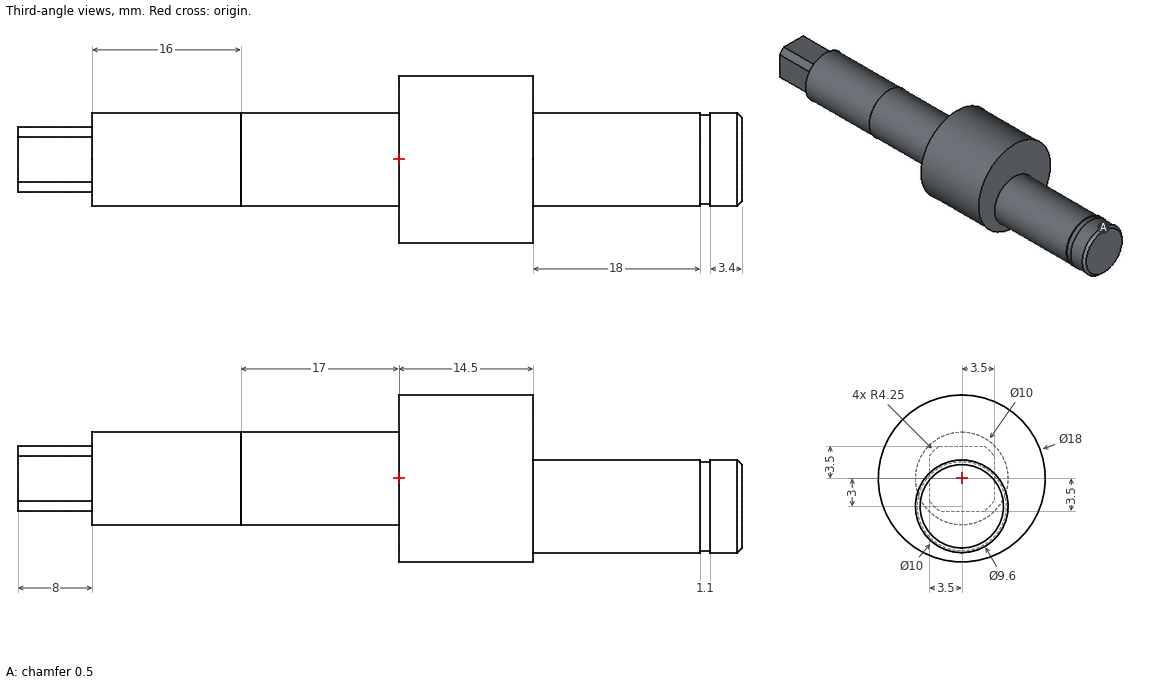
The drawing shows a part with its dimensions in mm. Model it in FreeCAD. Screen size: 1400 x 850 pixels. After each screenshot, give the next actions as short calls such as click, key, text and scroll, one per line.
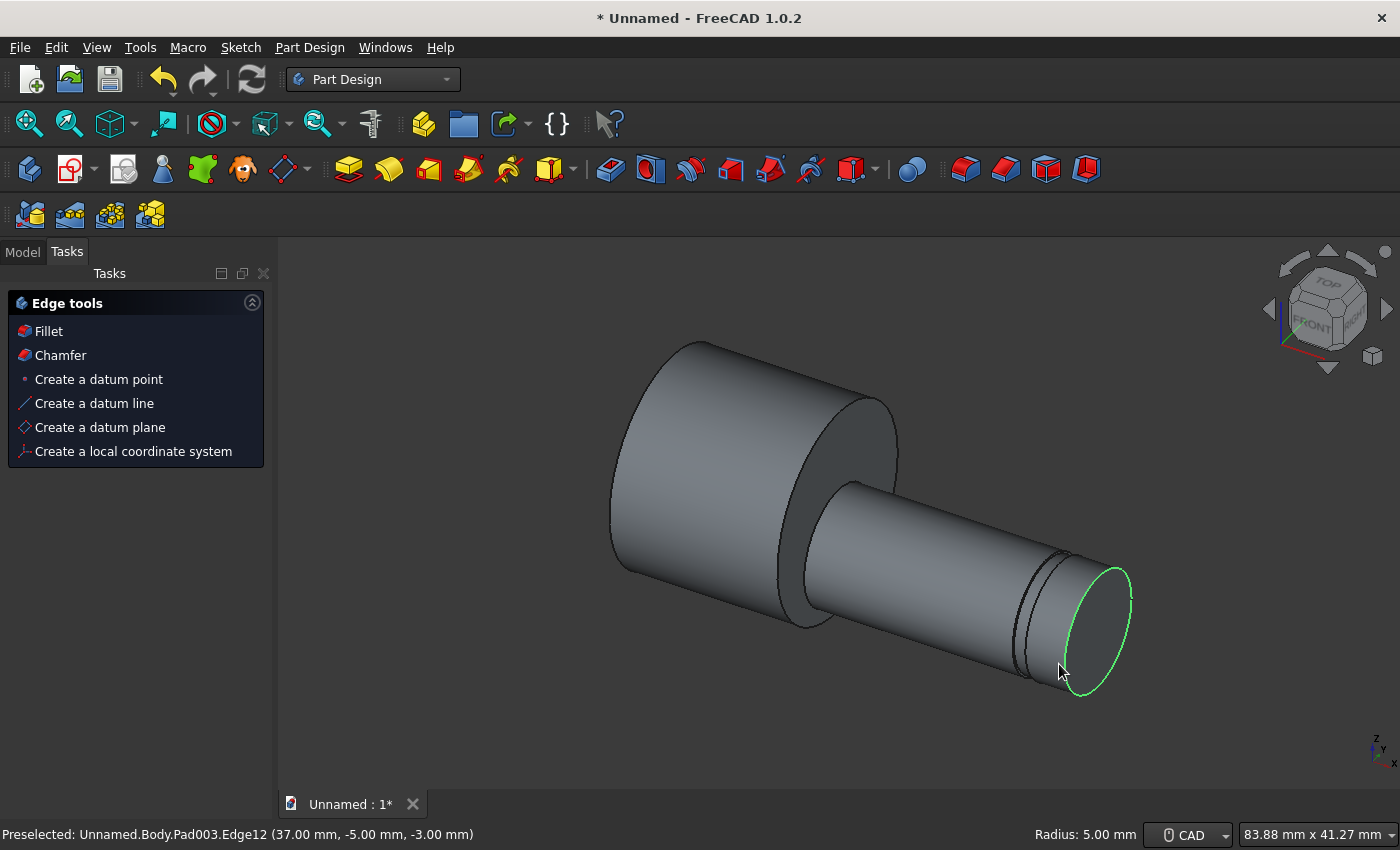
click(1006, 170)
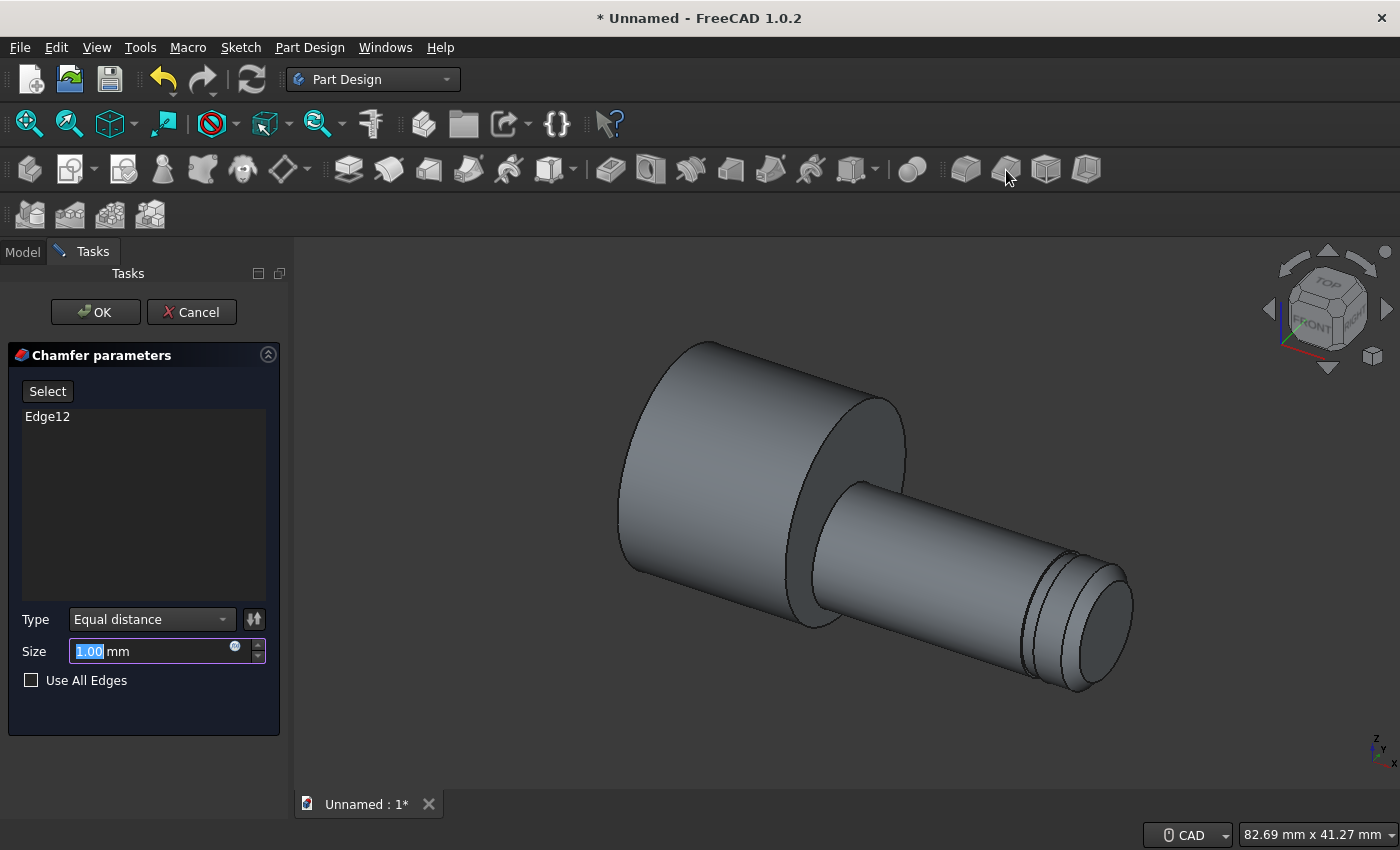
text(0.5)
key(Tab)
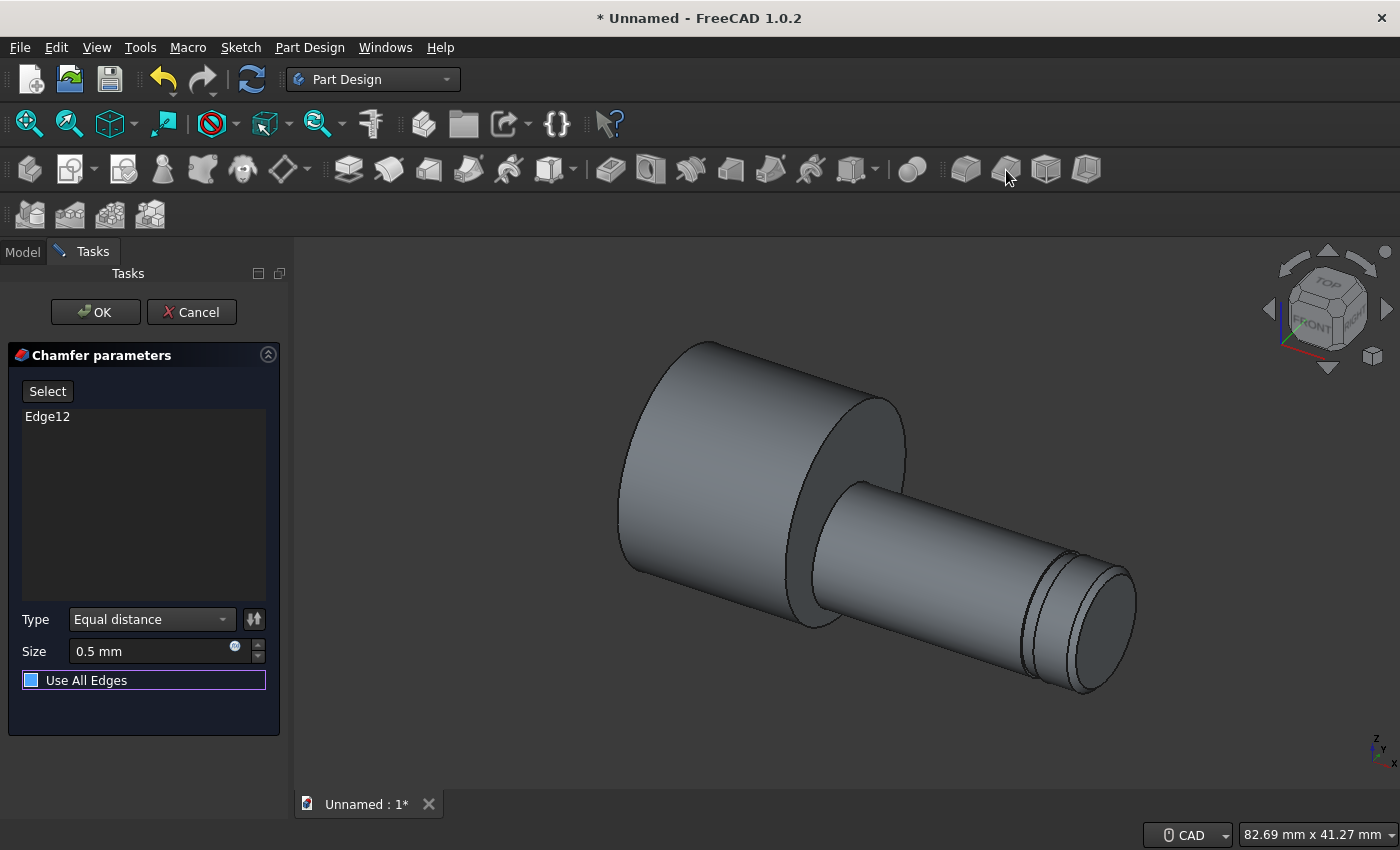
click(96, 312)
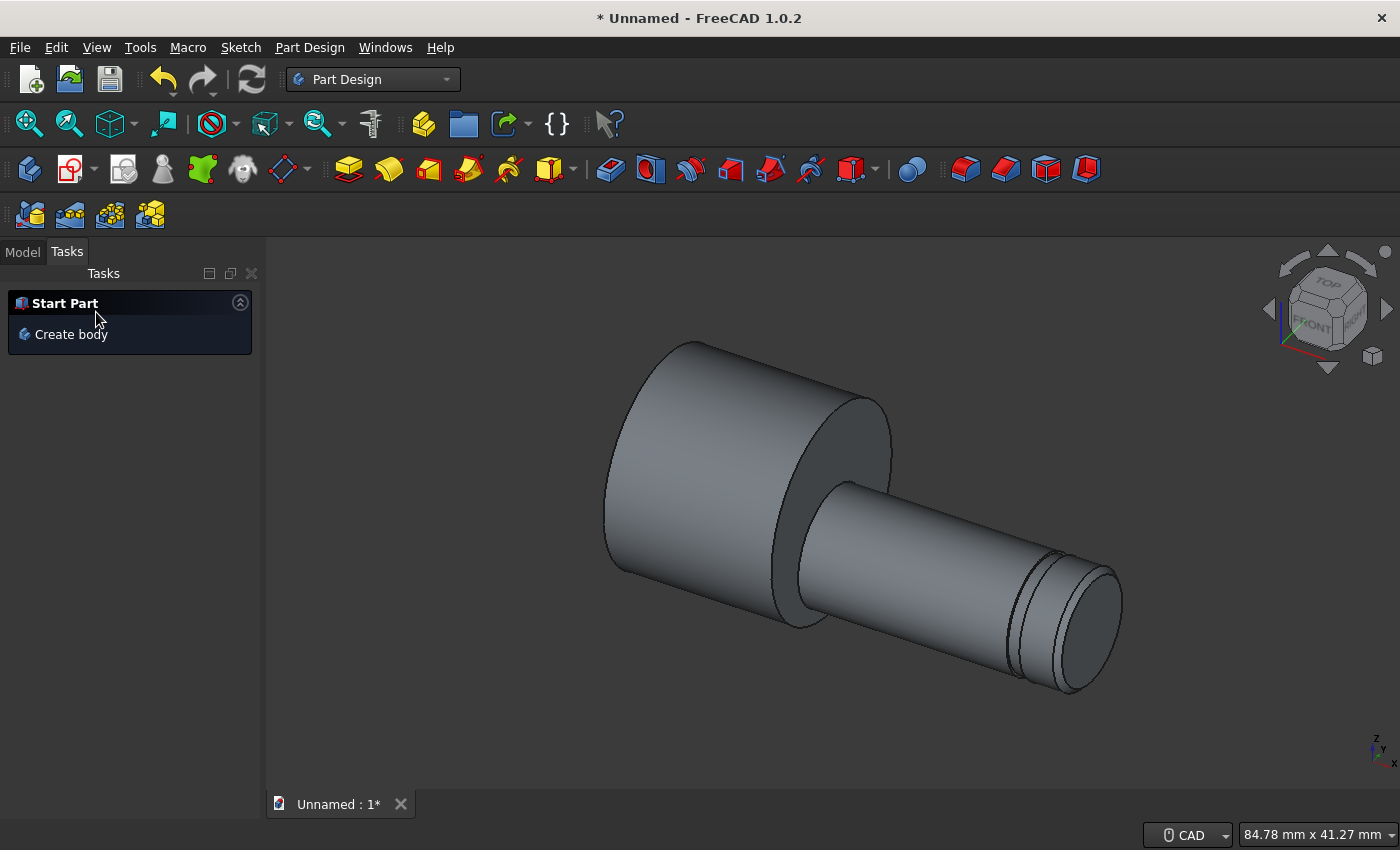
click(70, 170)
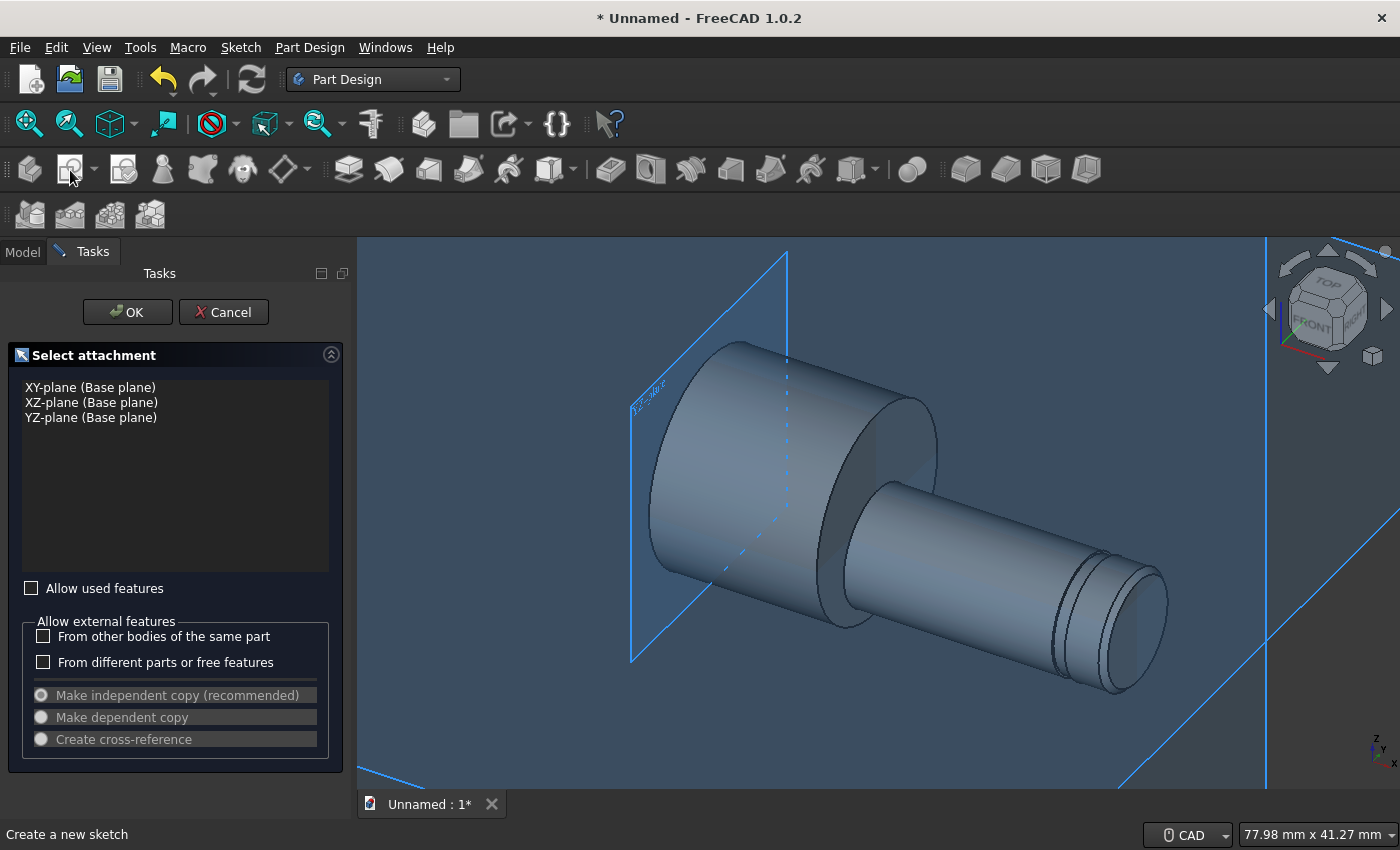
click(82, 418)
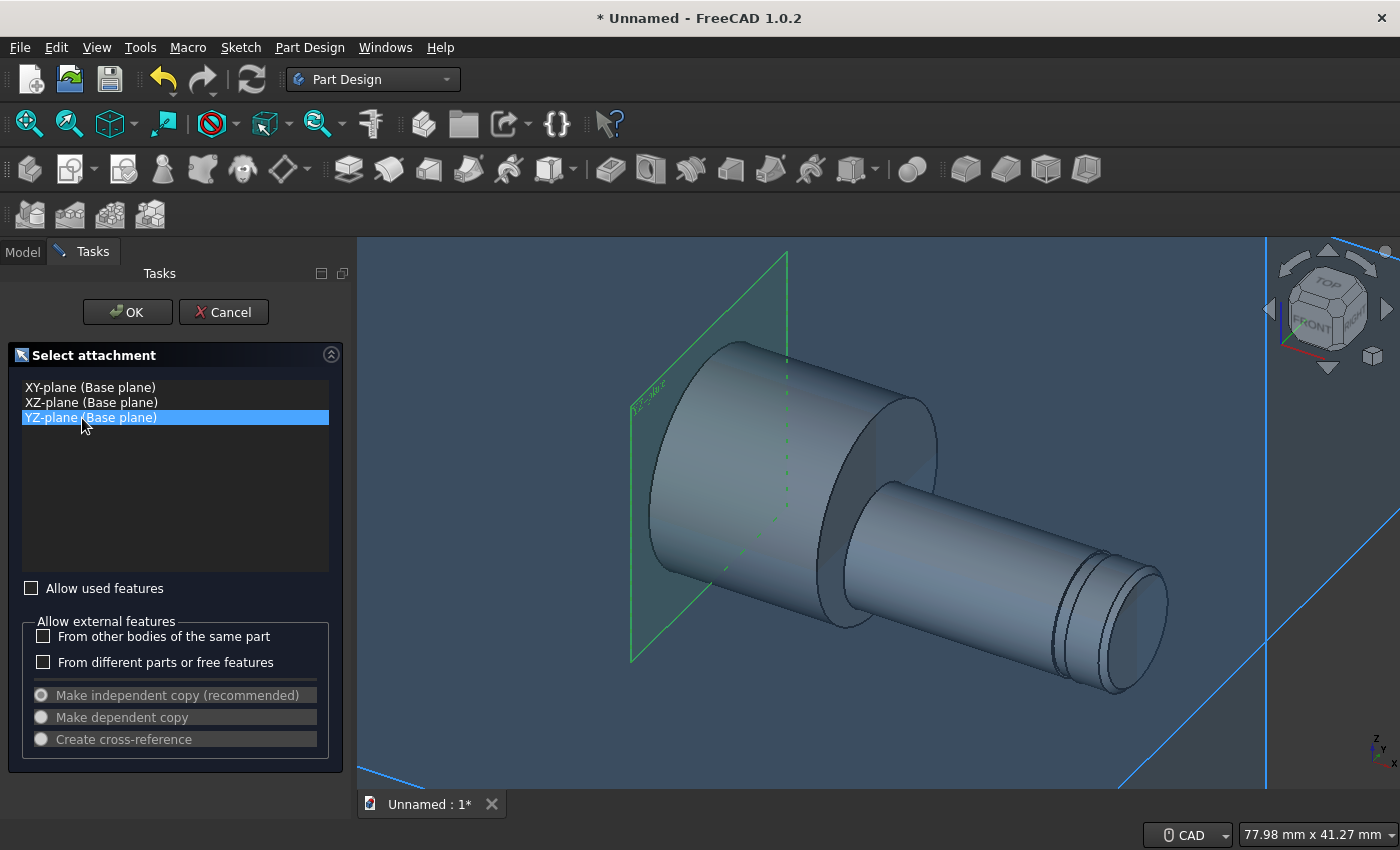
click(128, 312)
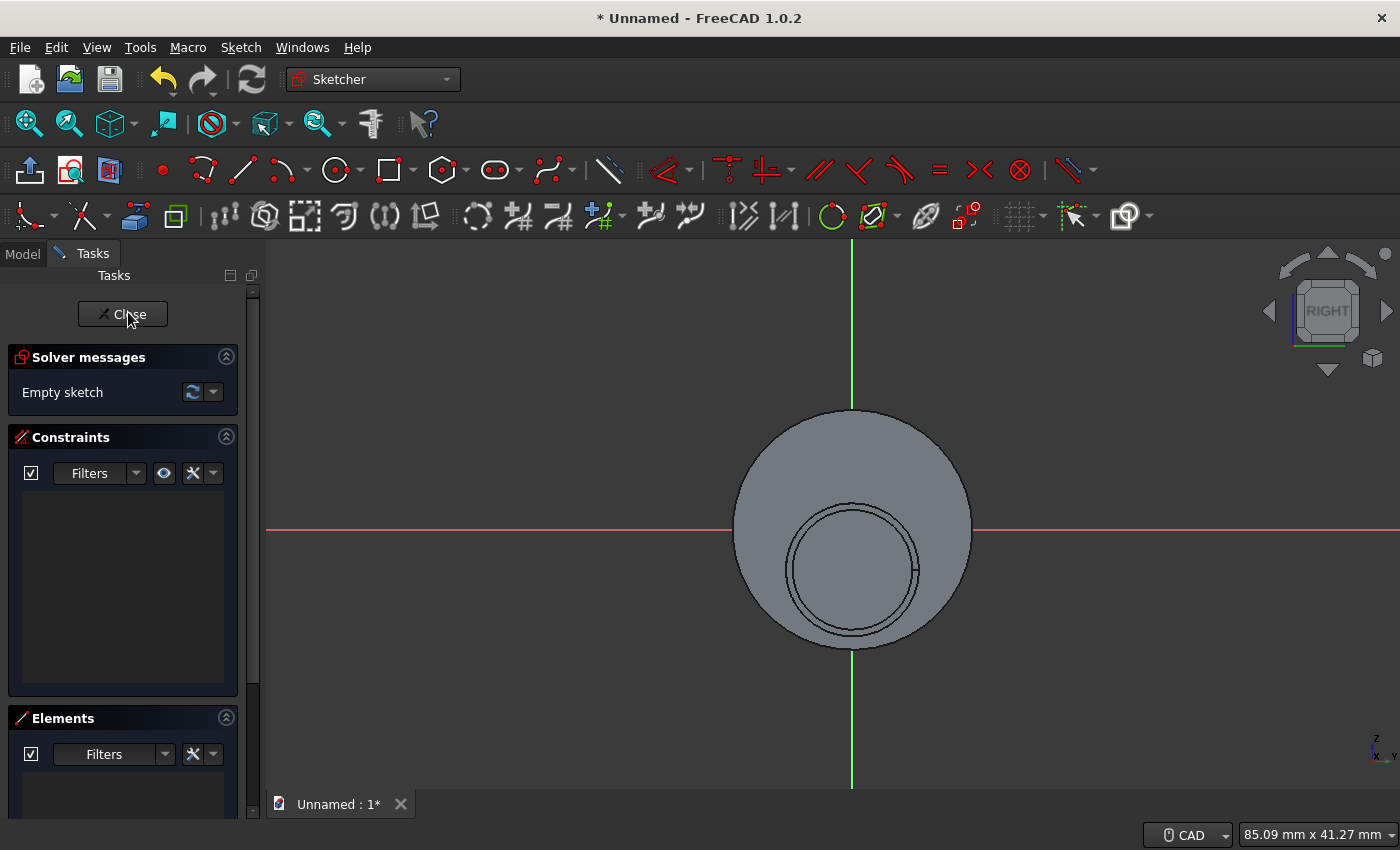
click(110, 170)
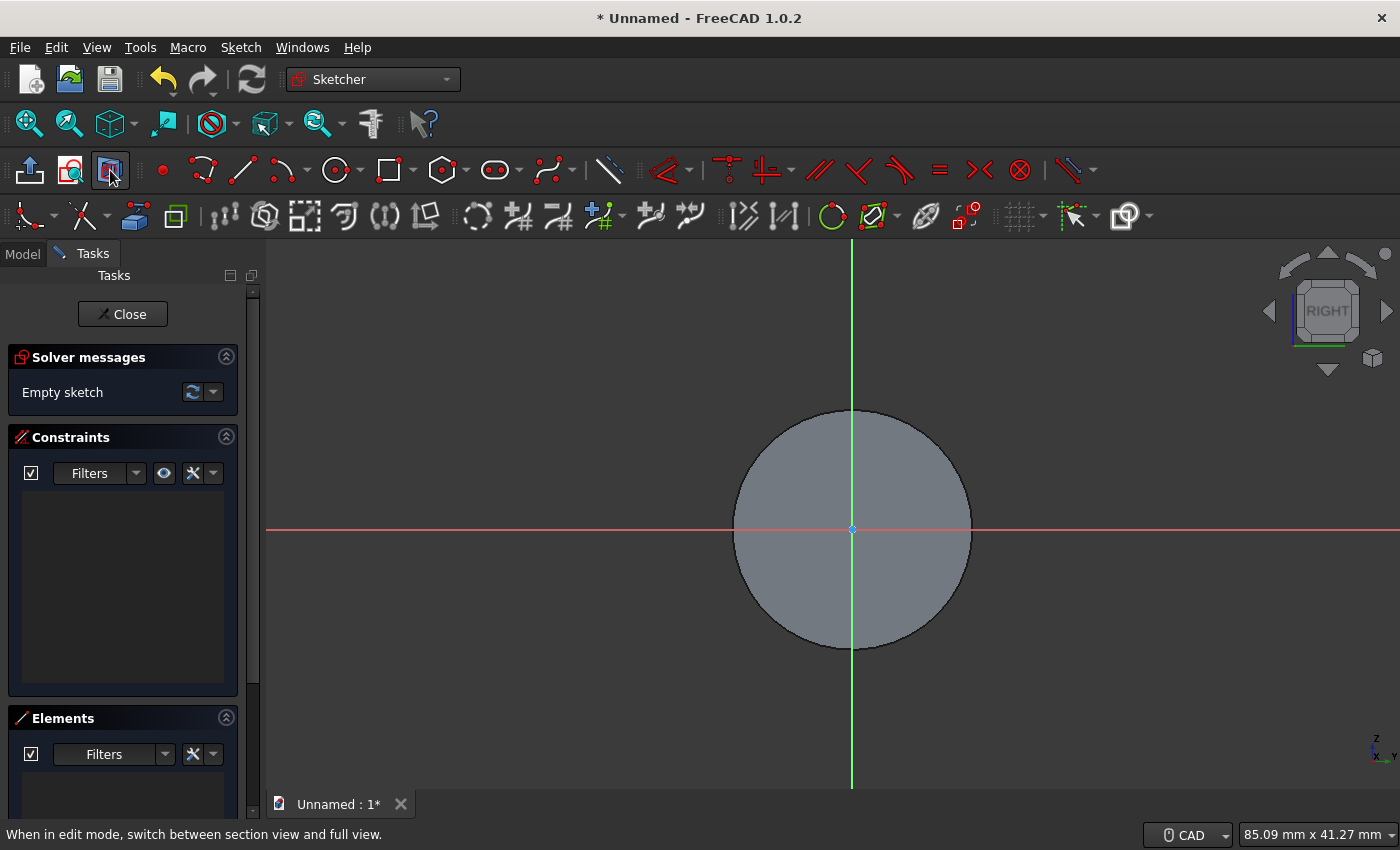
scroll(904, 539, up, 5)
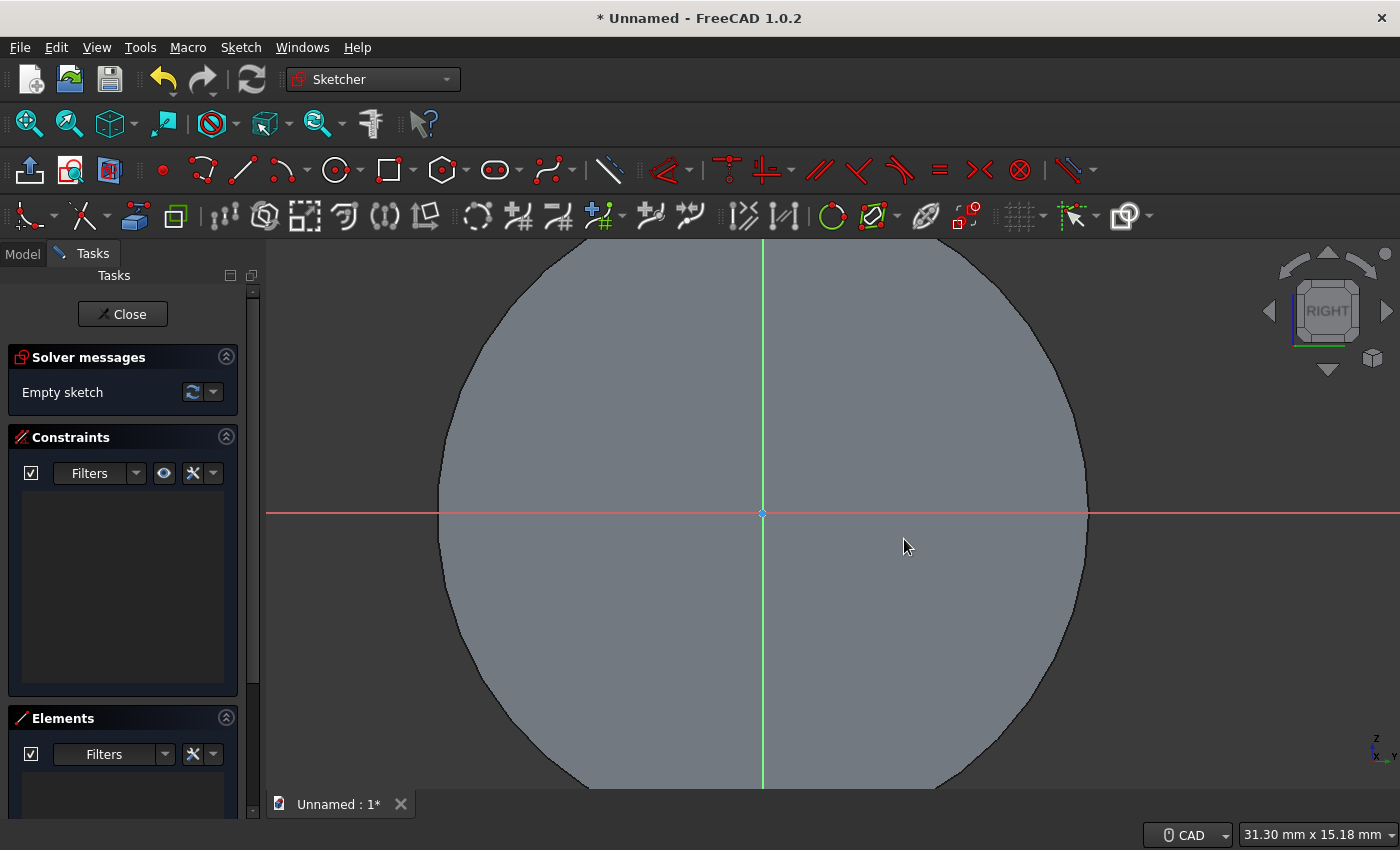
click(336, 170)